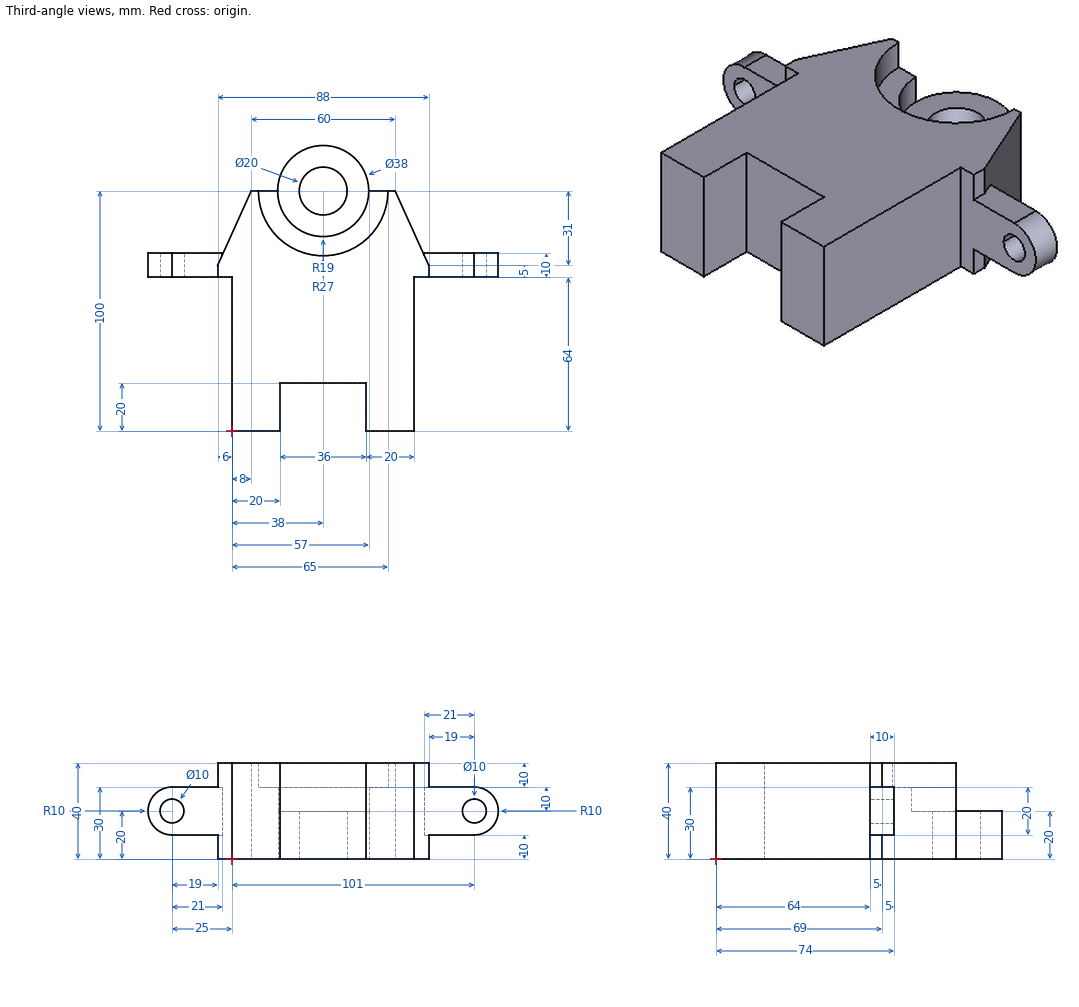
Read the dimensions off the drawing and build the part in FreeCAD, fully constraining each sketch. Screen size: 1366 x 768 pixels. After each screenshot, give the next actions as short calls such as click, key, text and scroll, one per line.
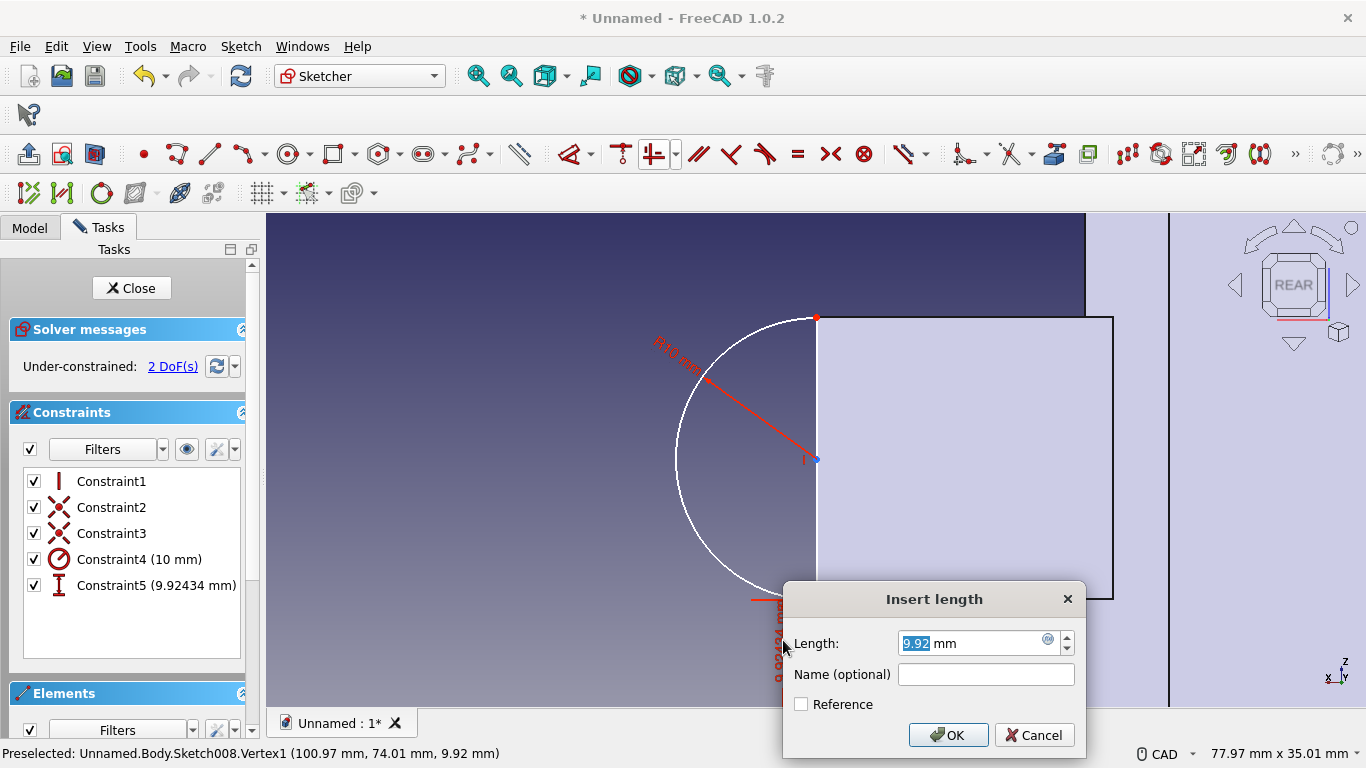
text(10)
key(Return)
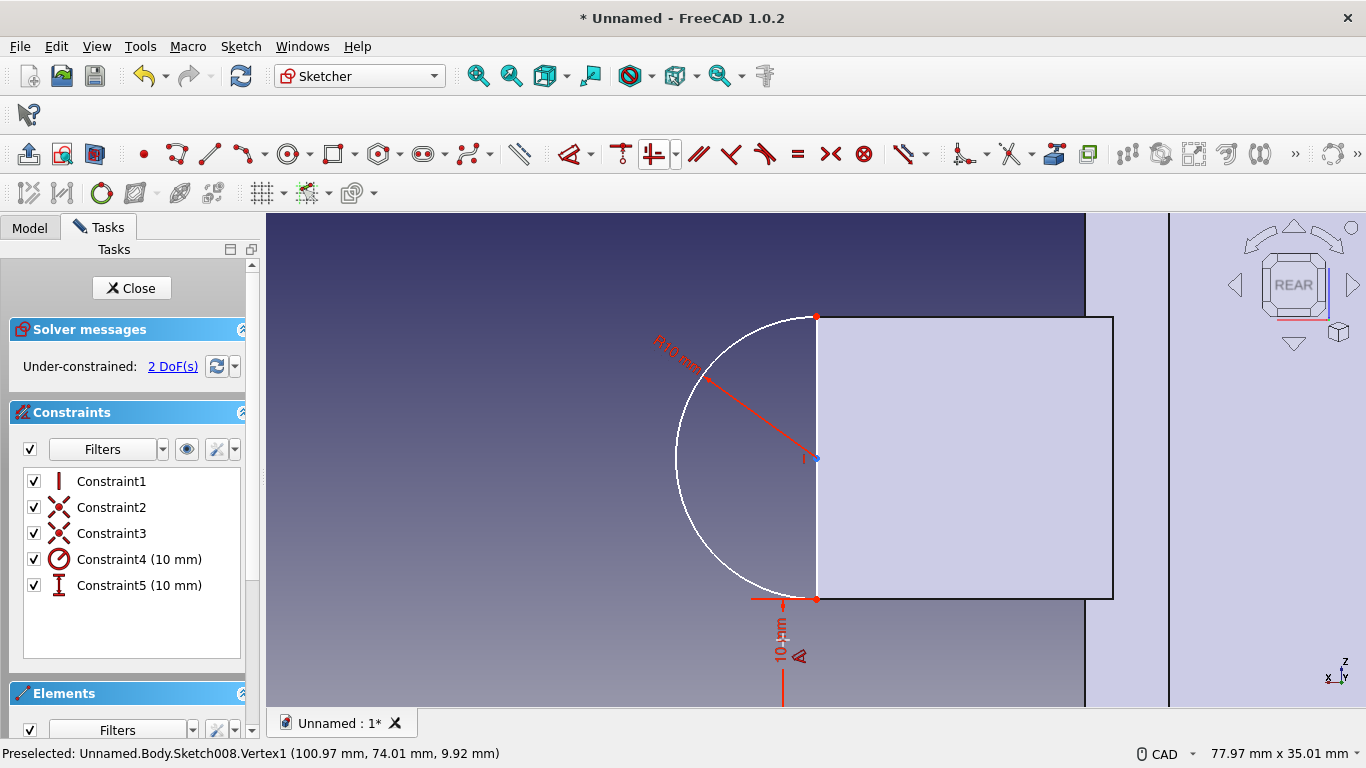
click(817, 599)
click(1009, 565)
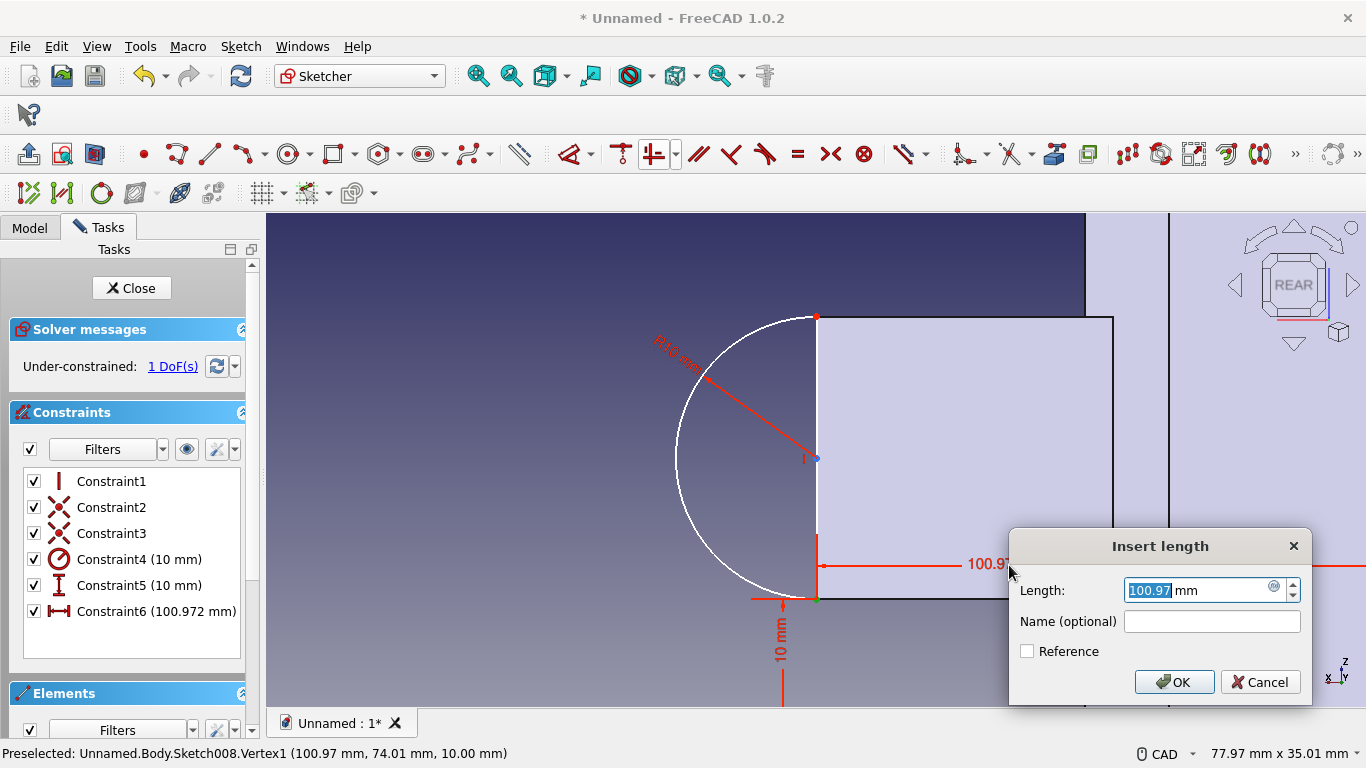
text(101)
key(Return)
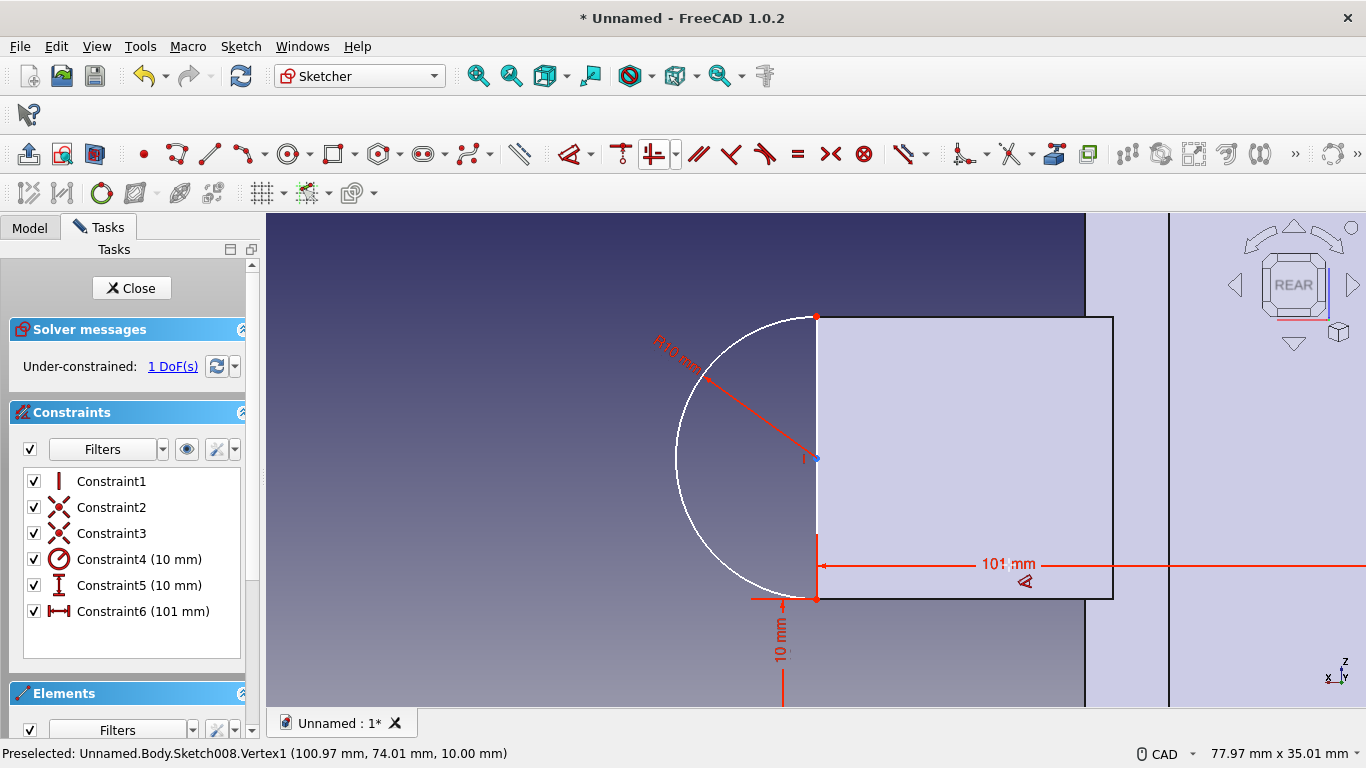
click(817, 458)
click(1009, 424)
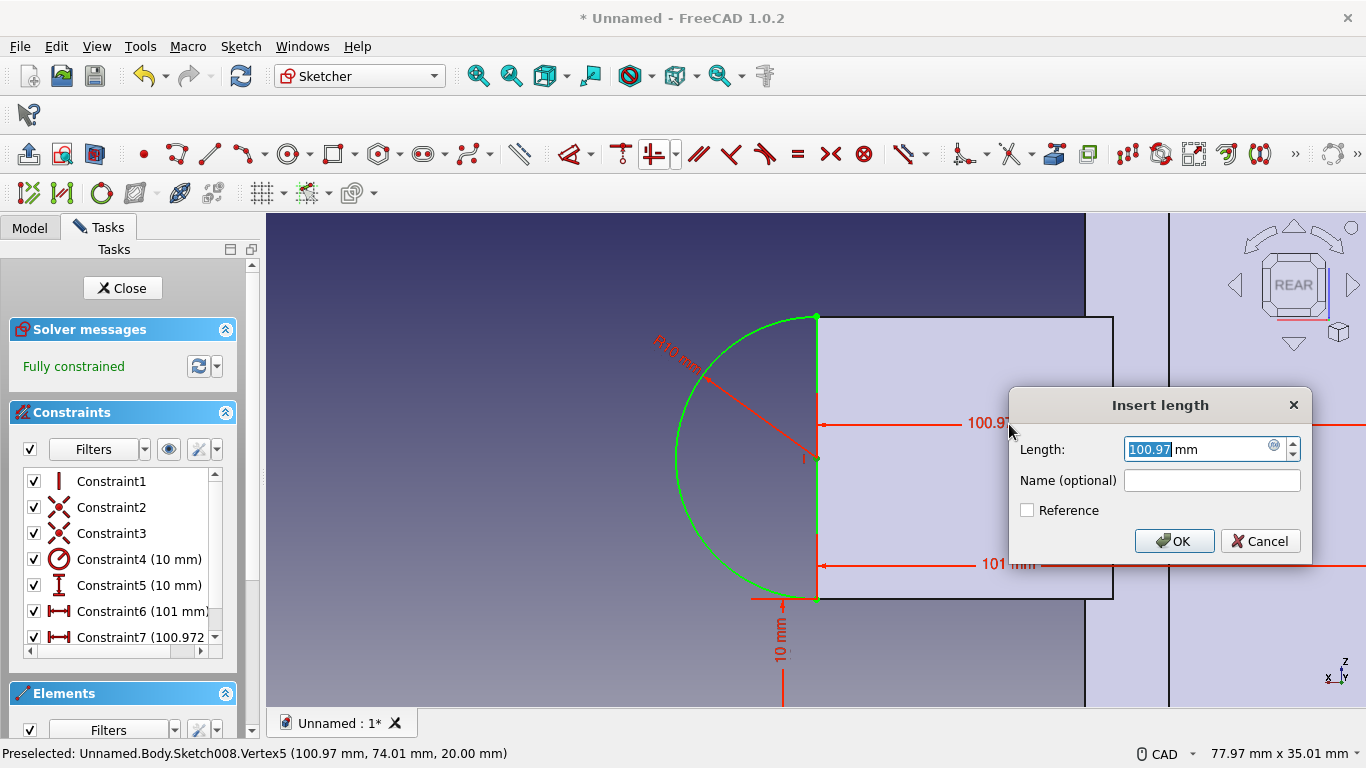
text(101)
key(Return)
key(Escape)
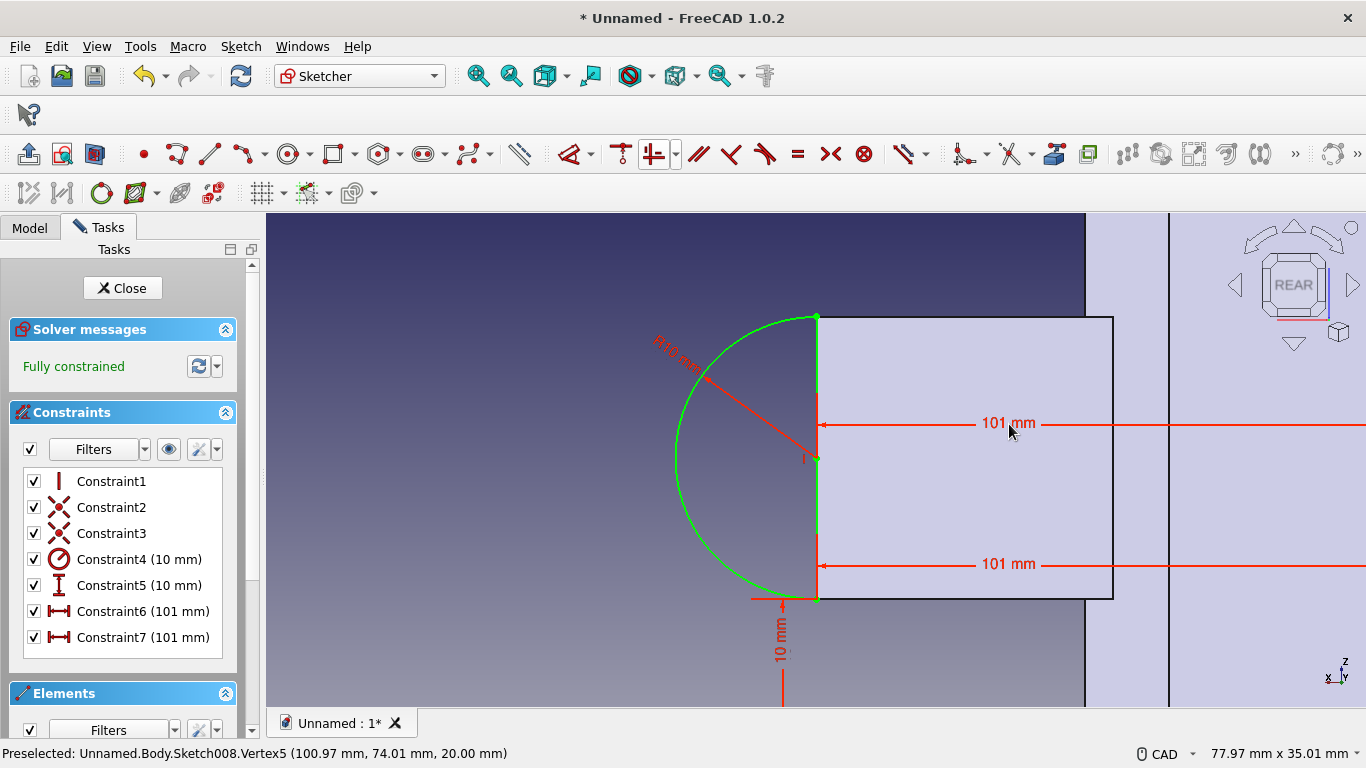
click(123, 288)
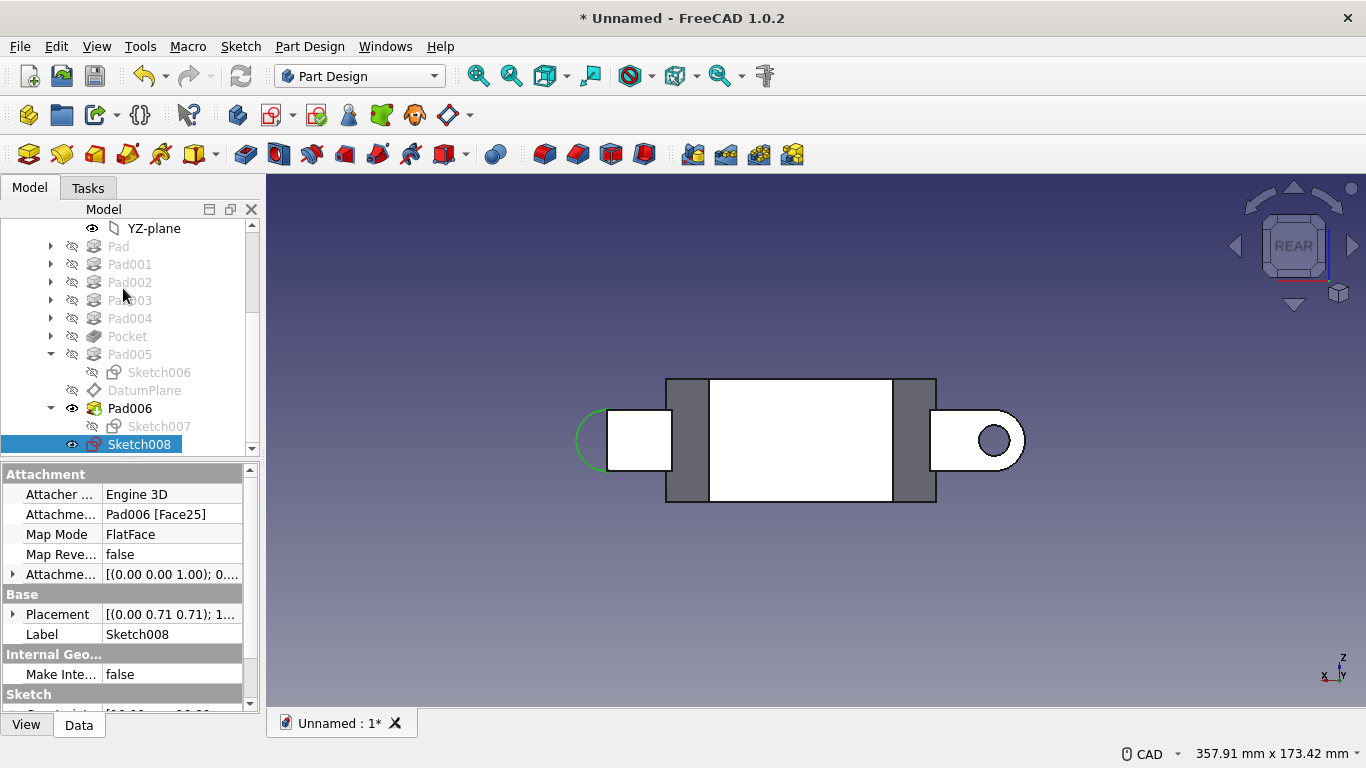
click(29, 154)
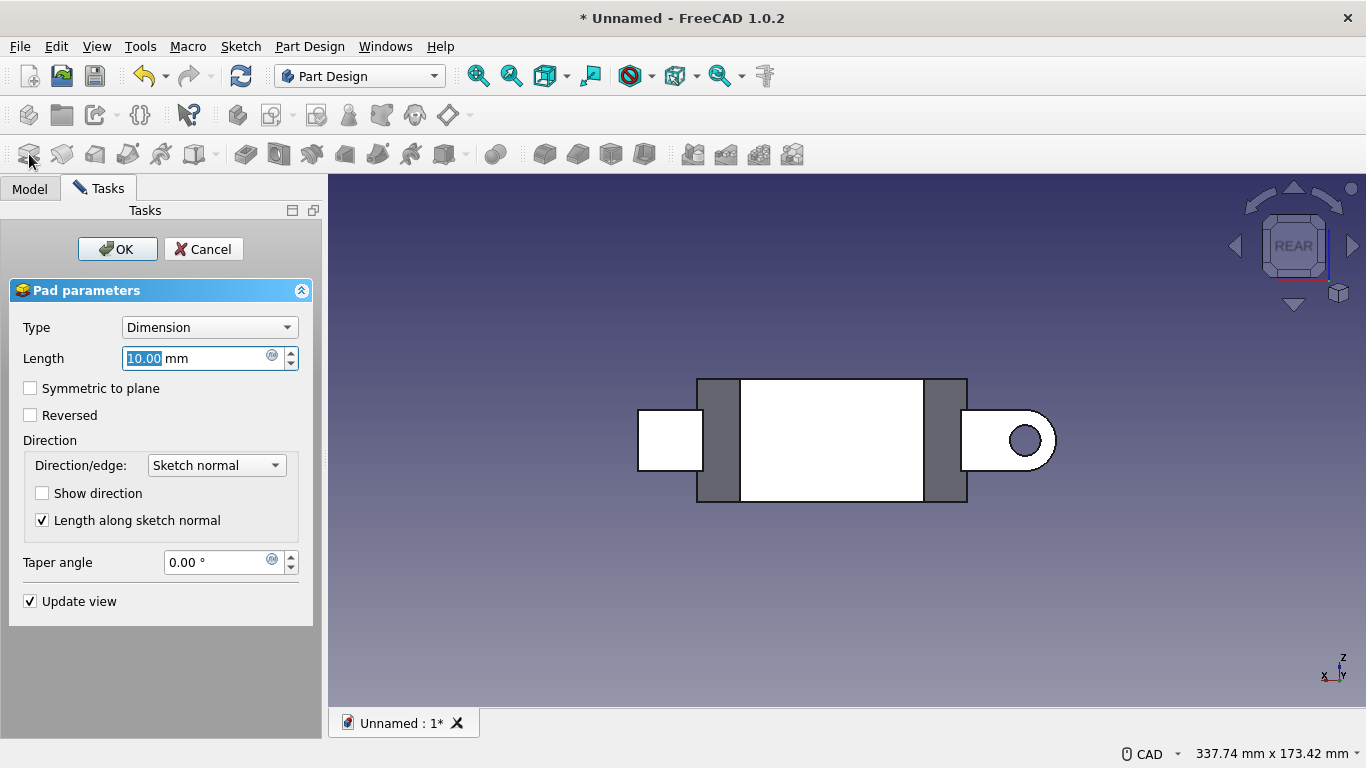
text(10)
key(Tab)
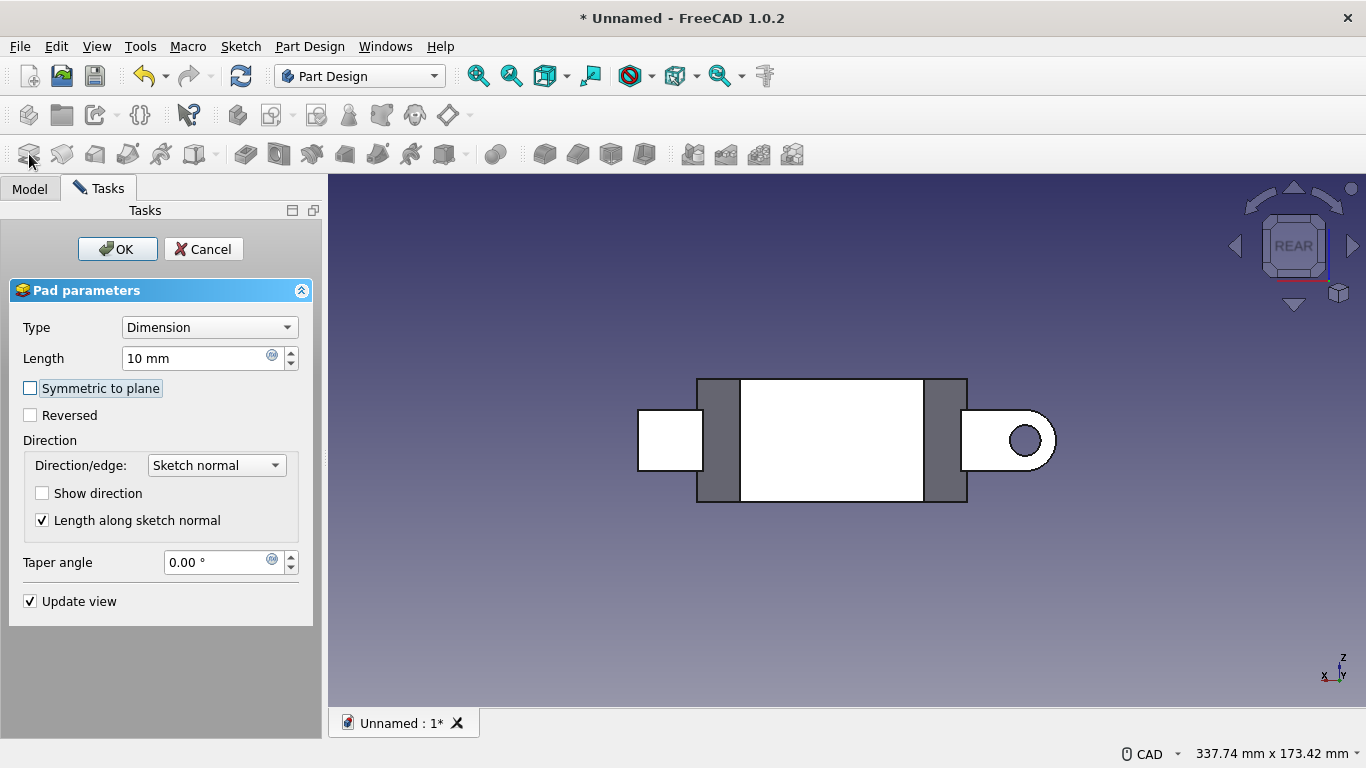
click(31, 415)